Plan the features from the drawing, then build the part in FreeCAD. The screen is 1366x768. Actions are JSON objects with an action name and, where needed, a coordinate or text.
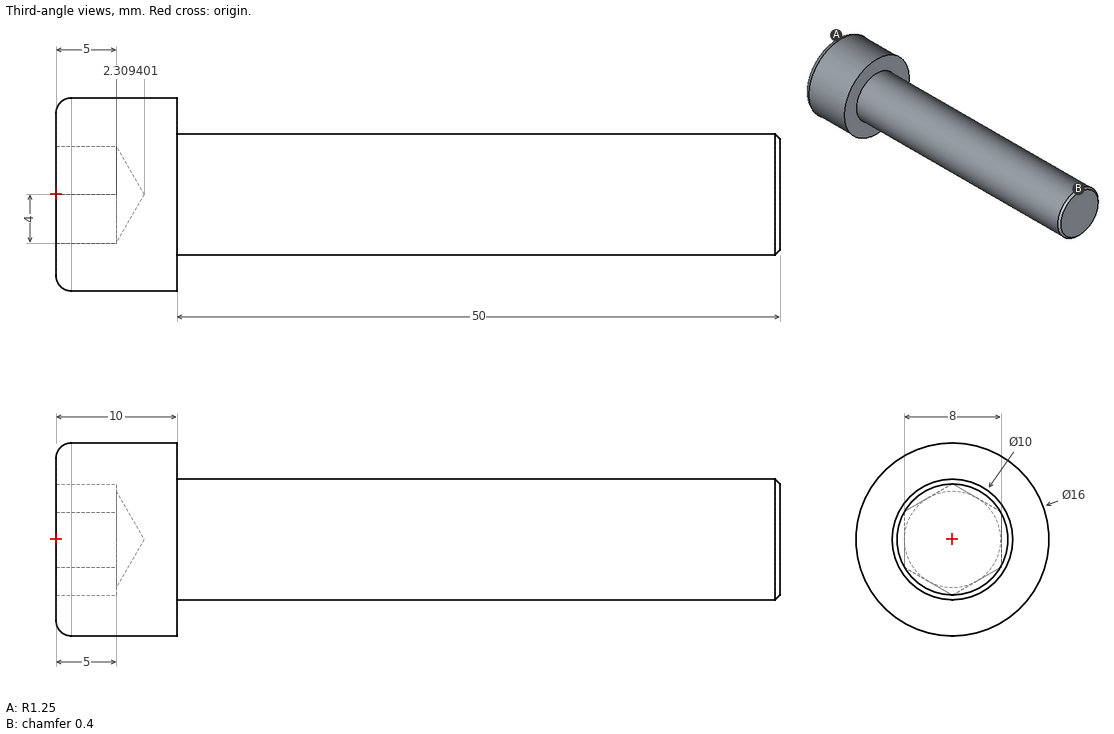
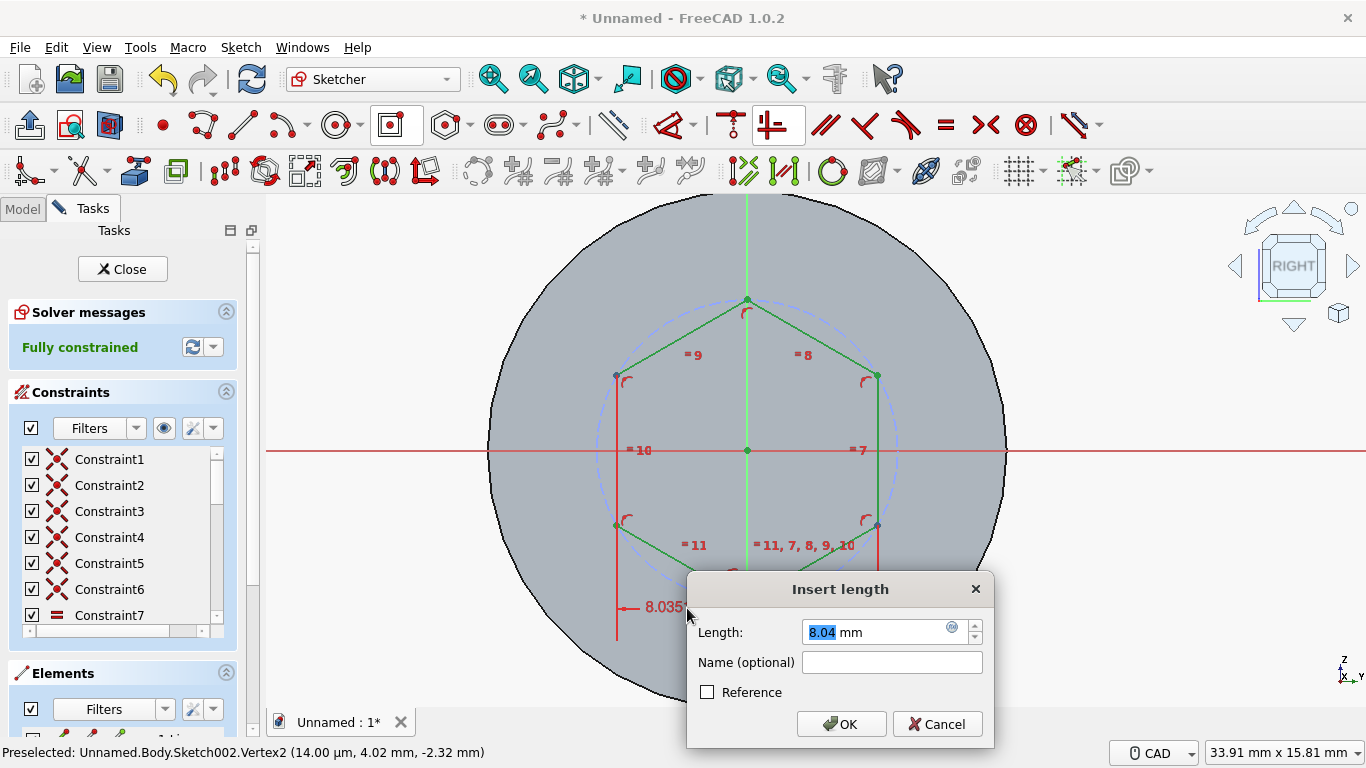
{"action": "type", "text": "8"}
{"action": "key", "text": "Return"}
{"action": "key", "text": "Escape"}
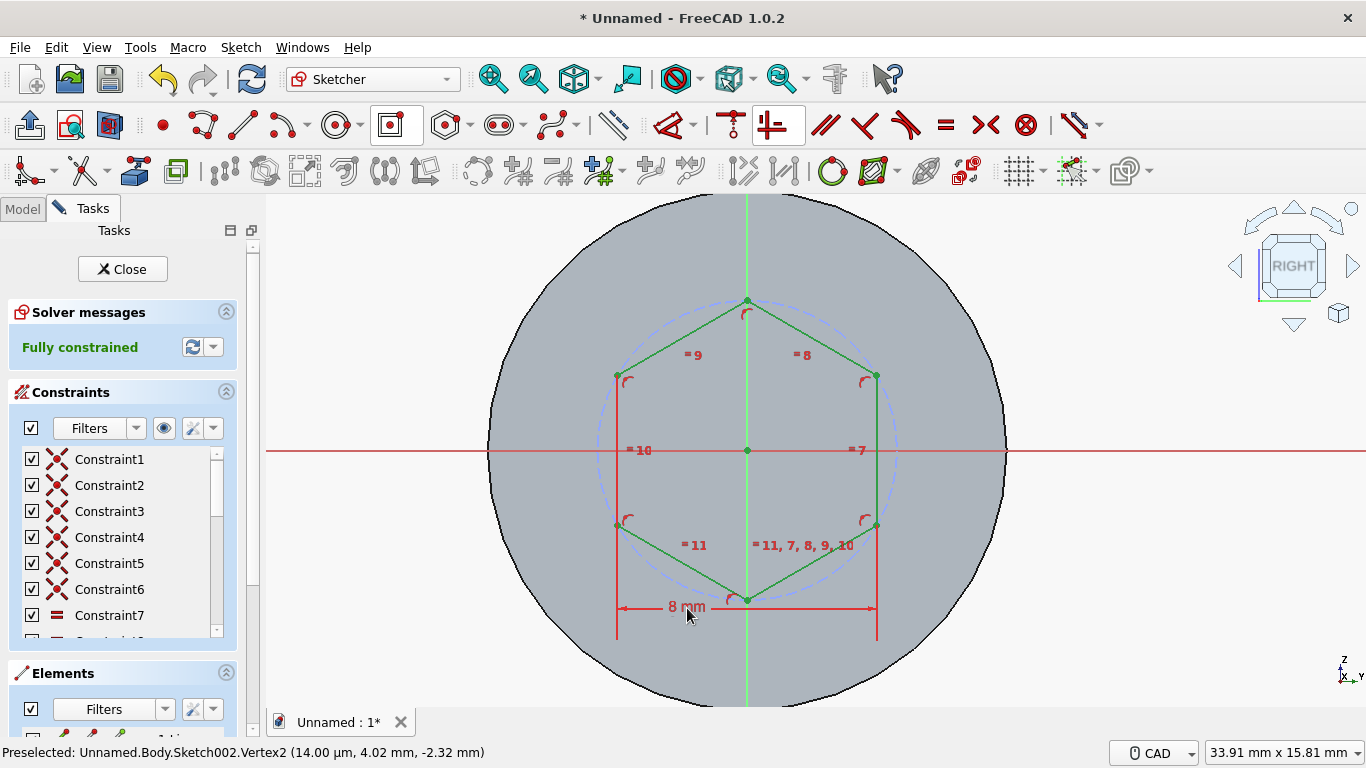
{"action": "left_click", "coordinate": [123, 269]}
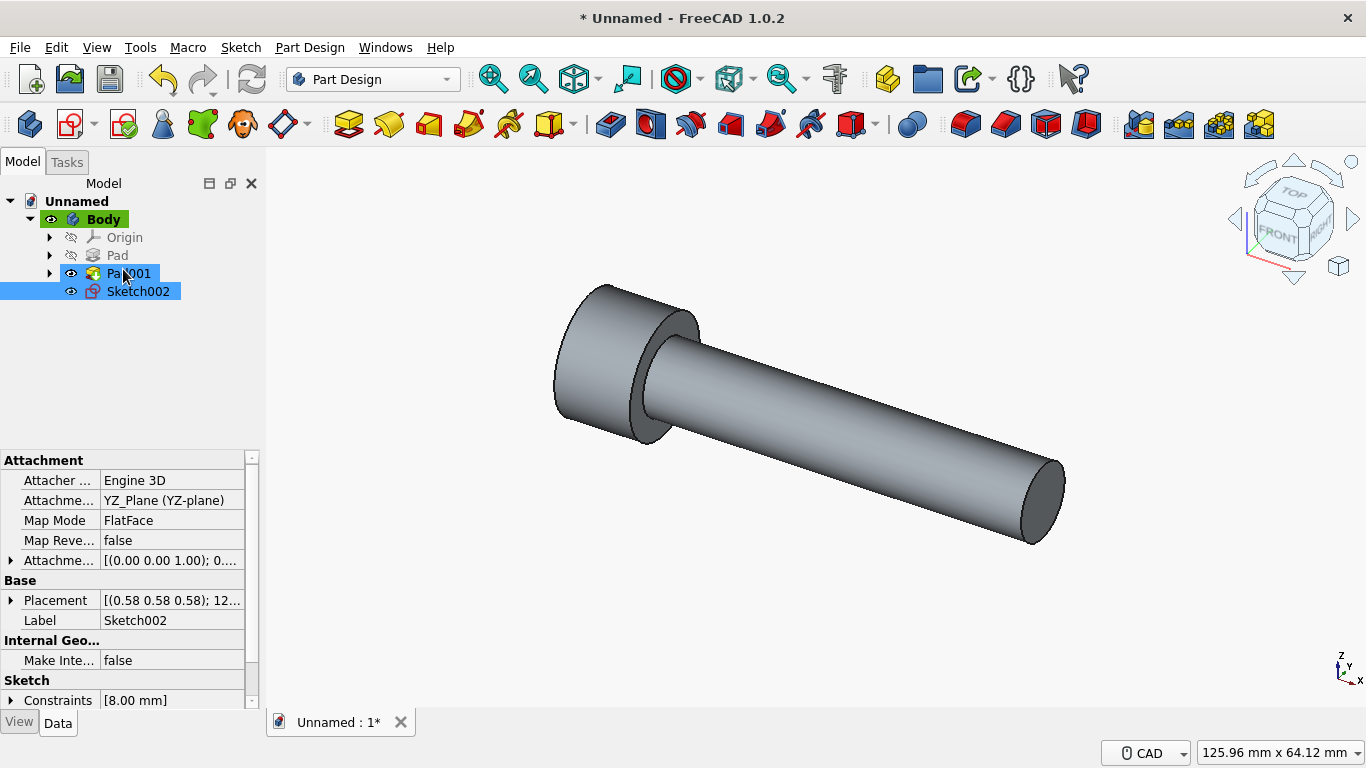
{"action": "left_click", "coordinate": [612, 124]}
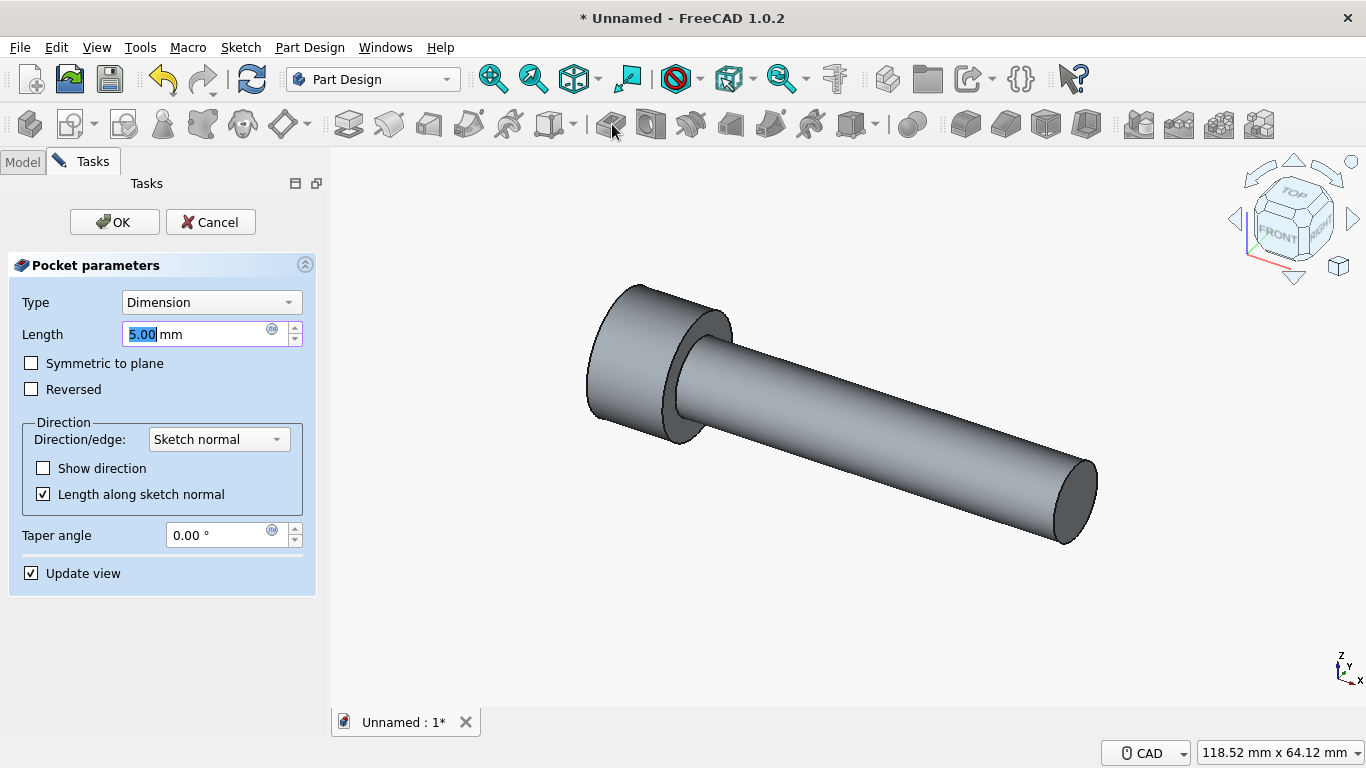
{"action": "type", "text": "5"}
{"action": "key", "text": "Tab"}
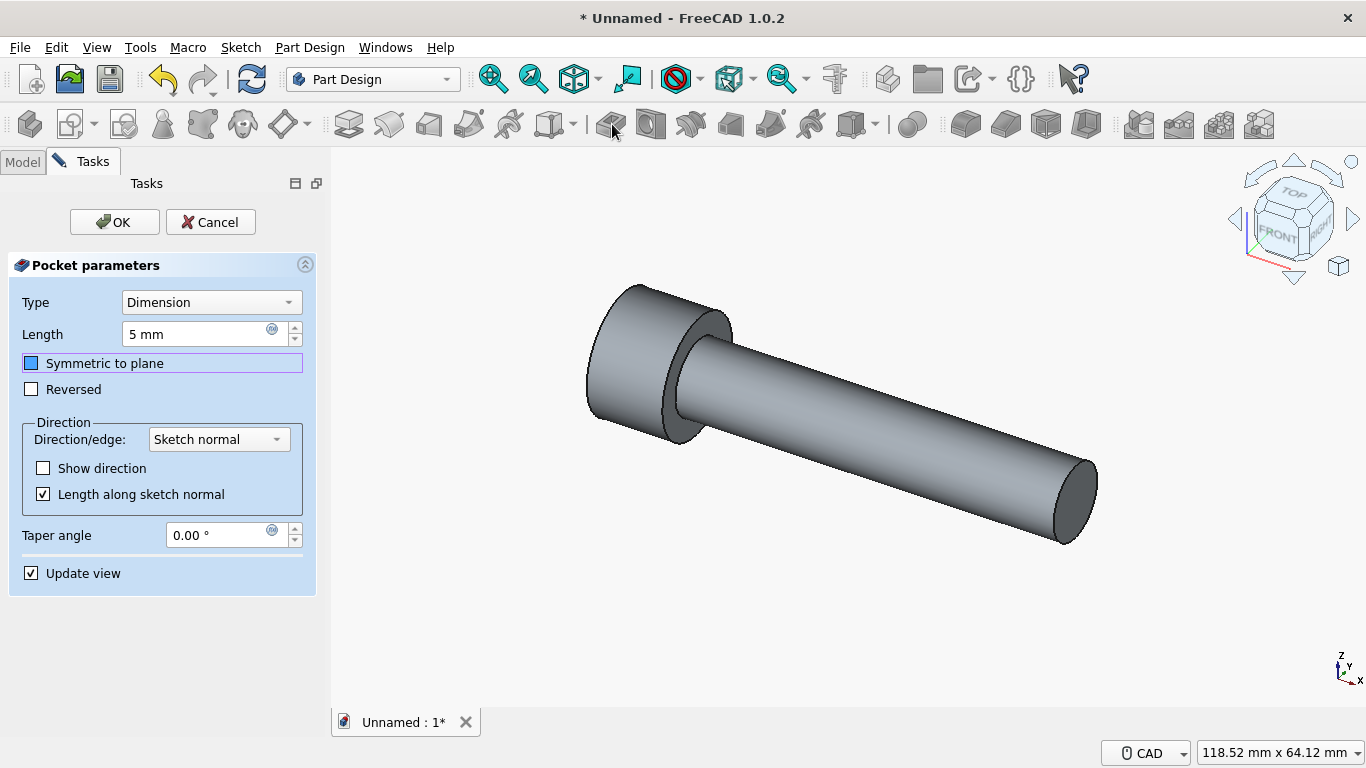
{"action": "left_click", "coordinate": [30, 389]}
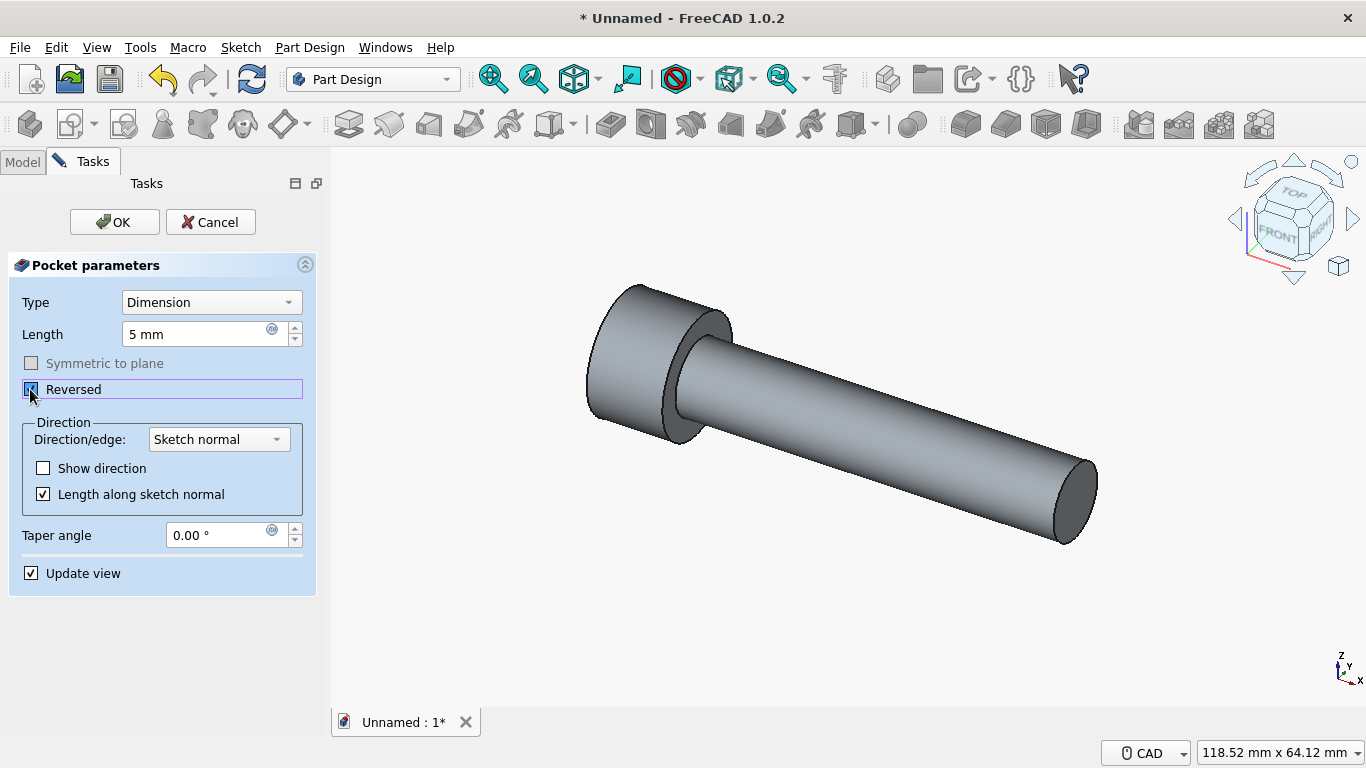
{"action": "left_click", "coordinate": [115, 222]}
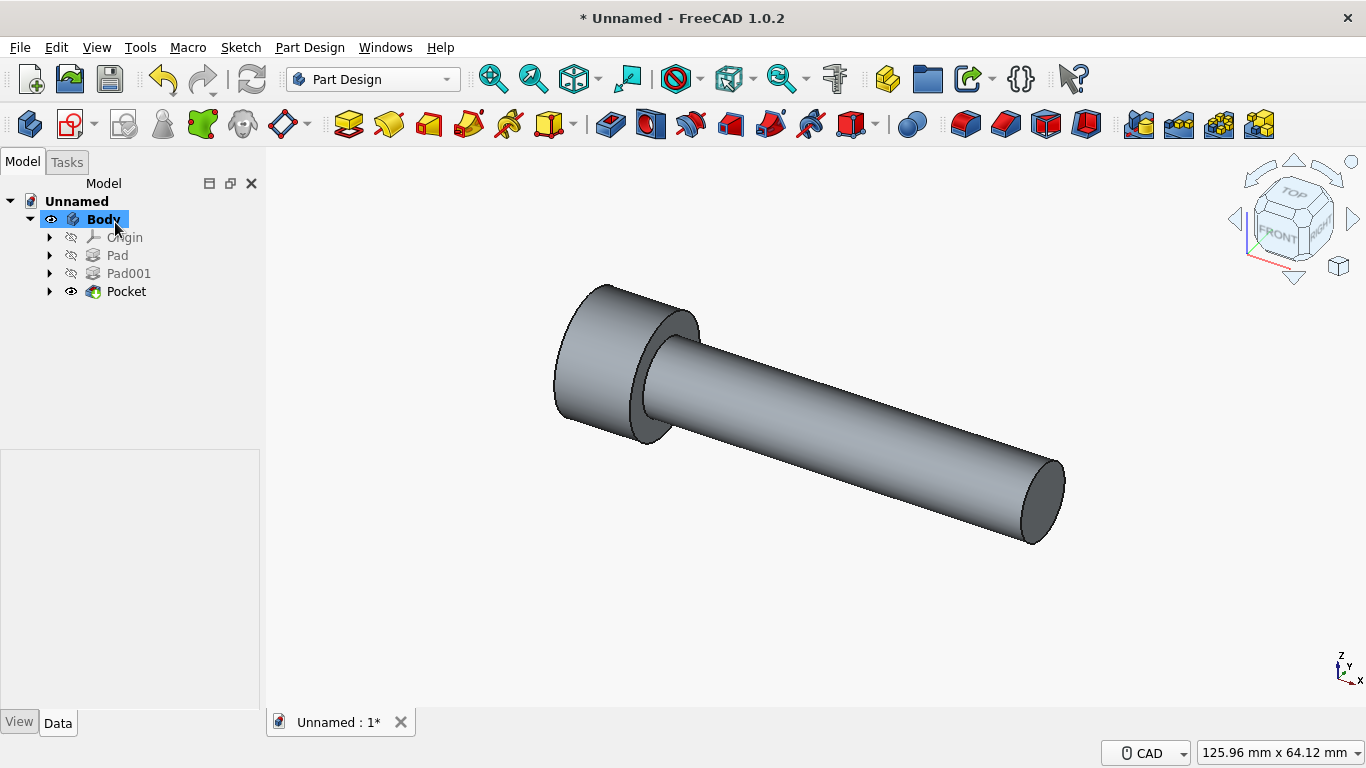
{"action": "left_click", "coordinate": [70, 124]}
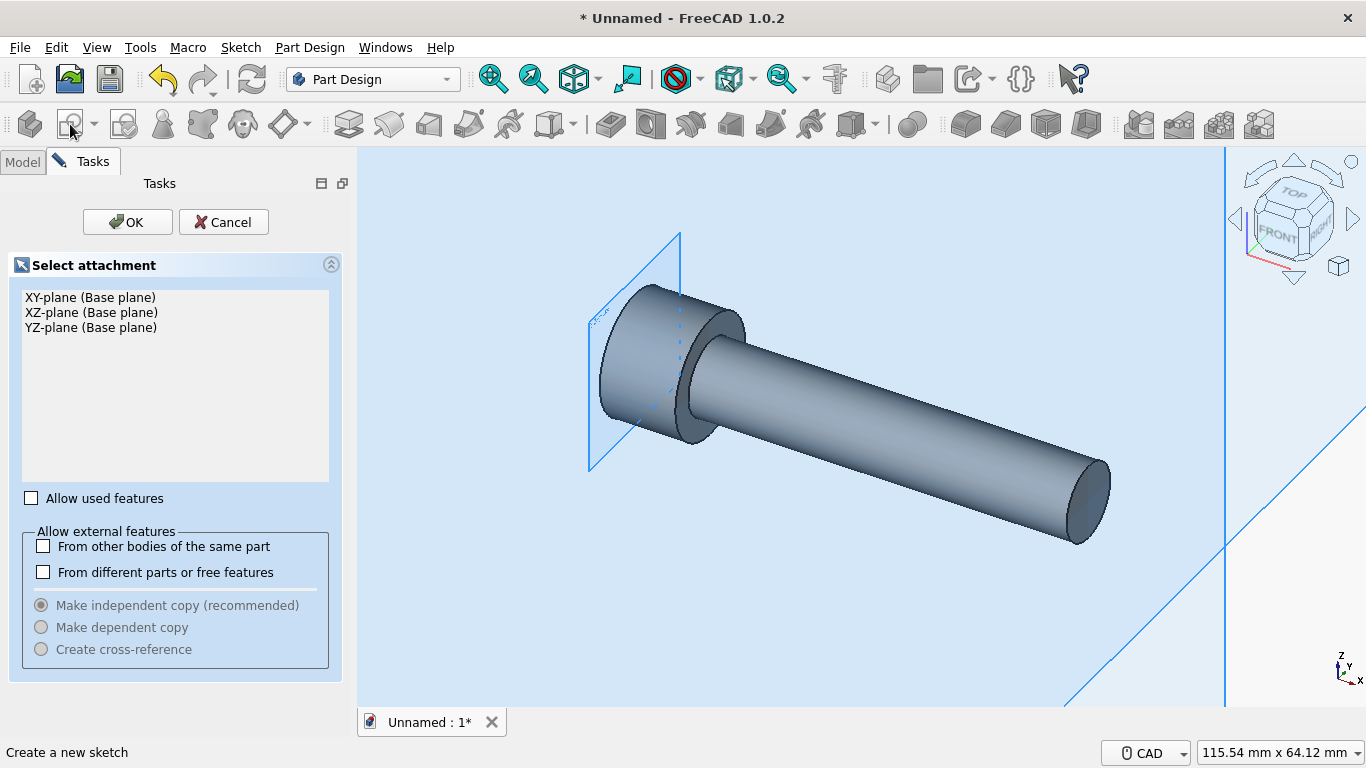
{"action": "left_click", "coordinate": [82, 298]}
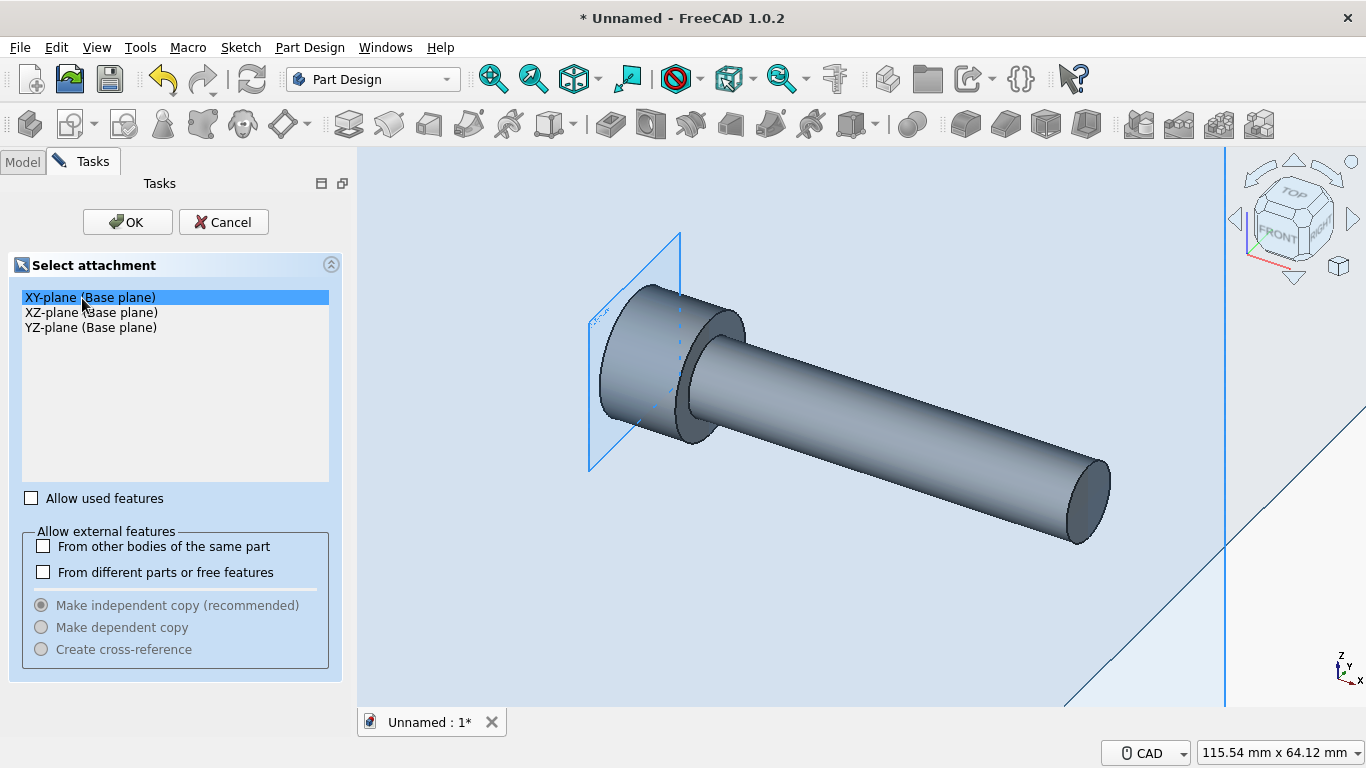
{"action": "left_click", "coordinate": [128, 222]}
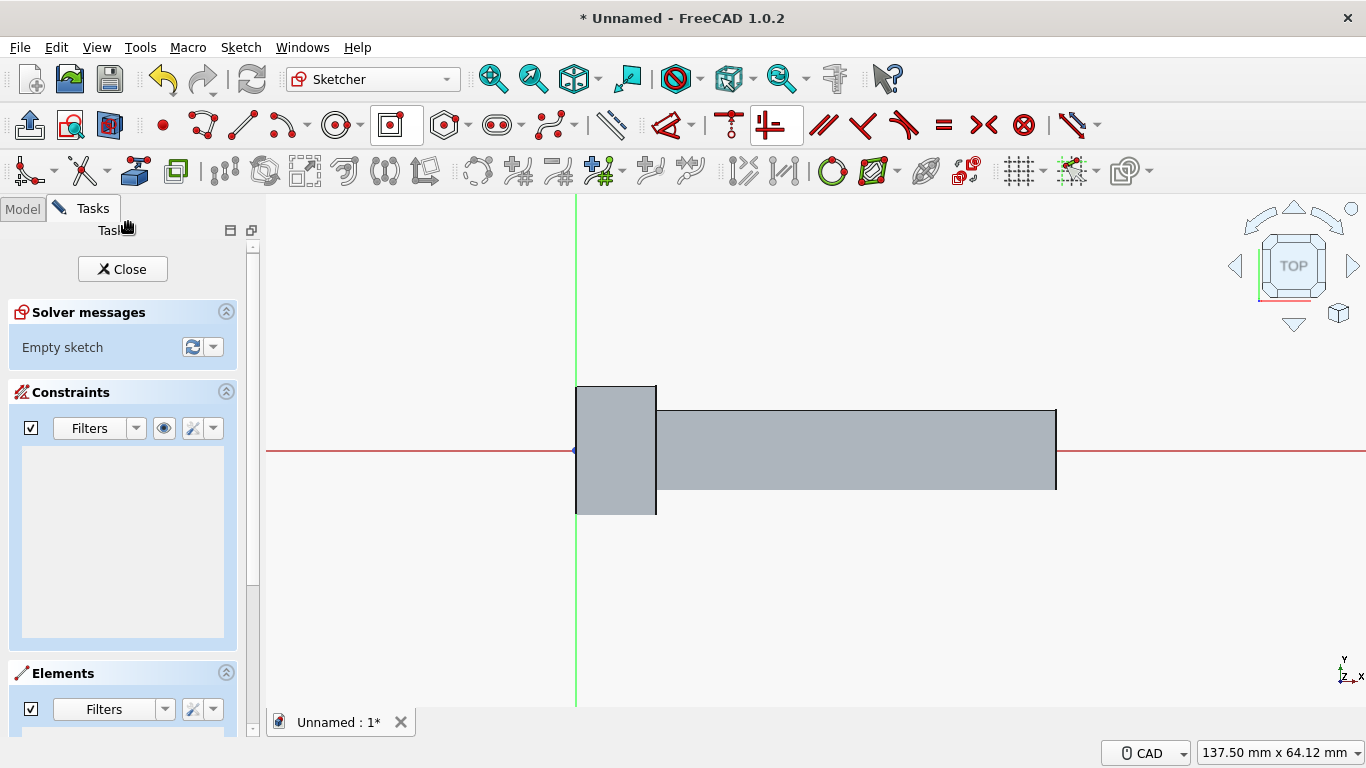
{"action": "left_click", "coordinate": [110, 126]}